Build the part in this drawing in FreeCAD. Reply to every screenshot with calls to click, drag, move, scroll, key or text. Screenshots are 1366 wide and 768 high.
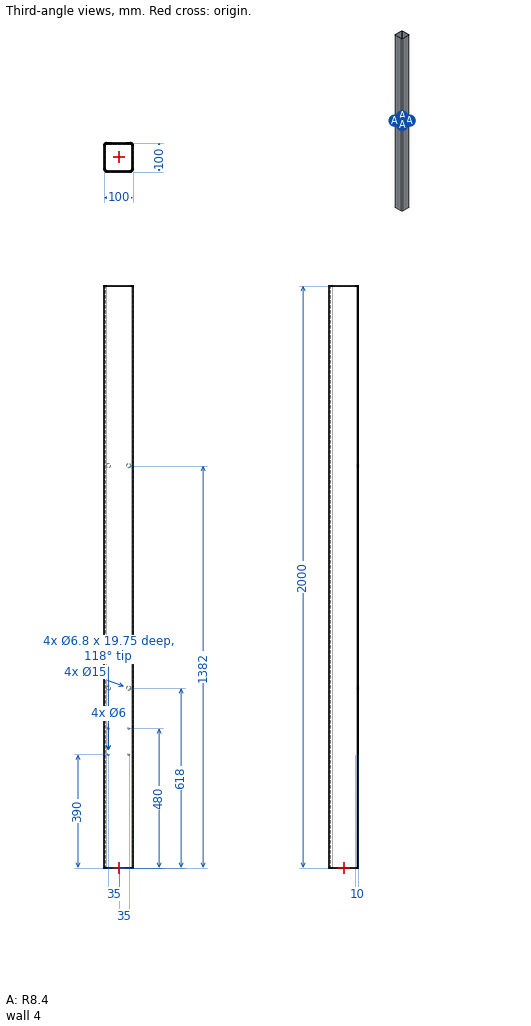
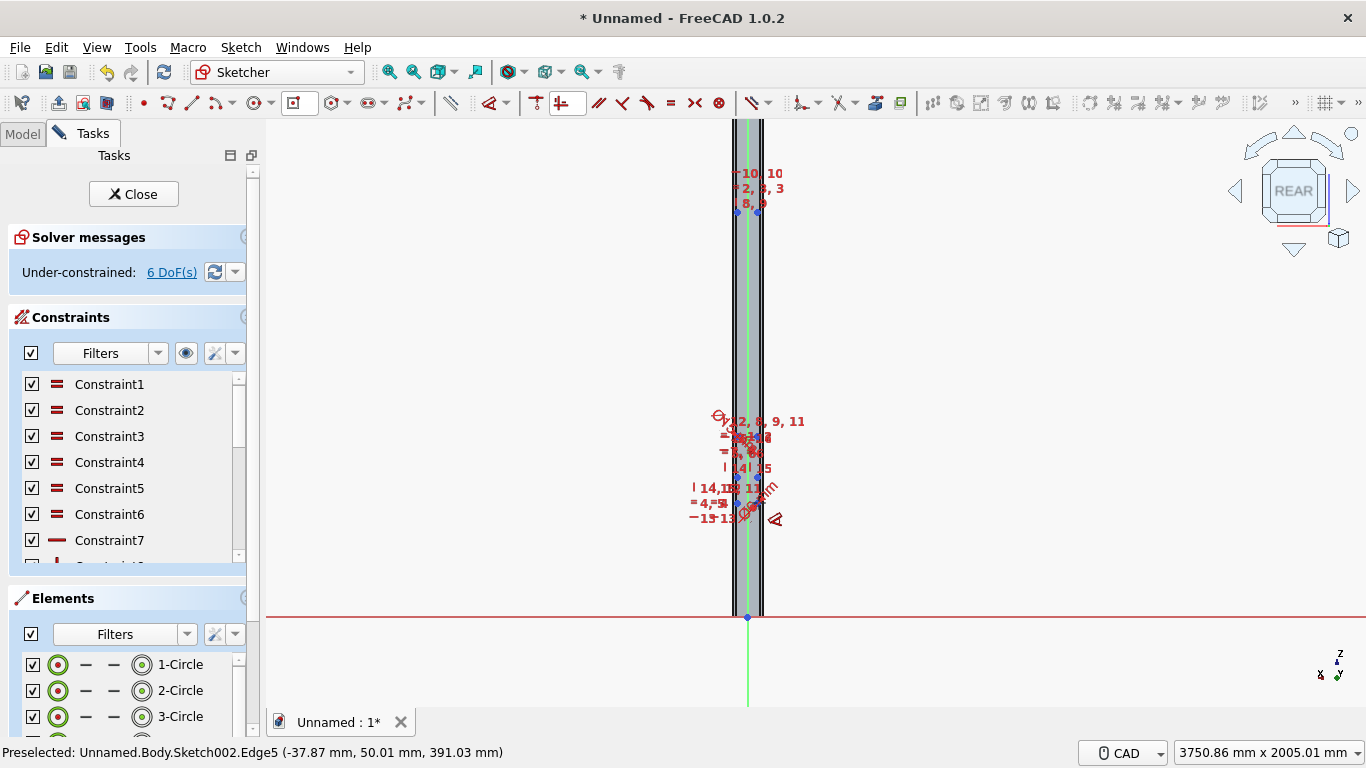
scroll(738, 437, up, 7)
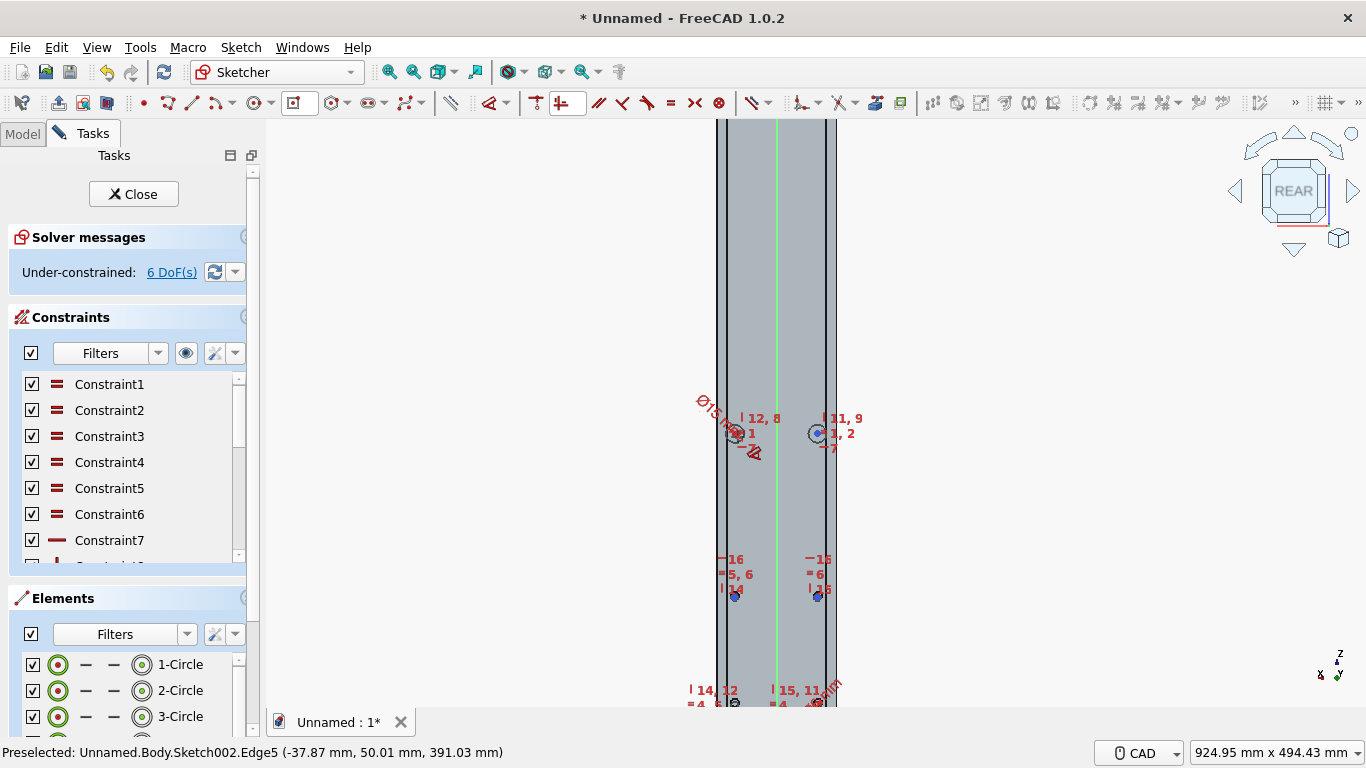
click(735, 434)
click(756, 376)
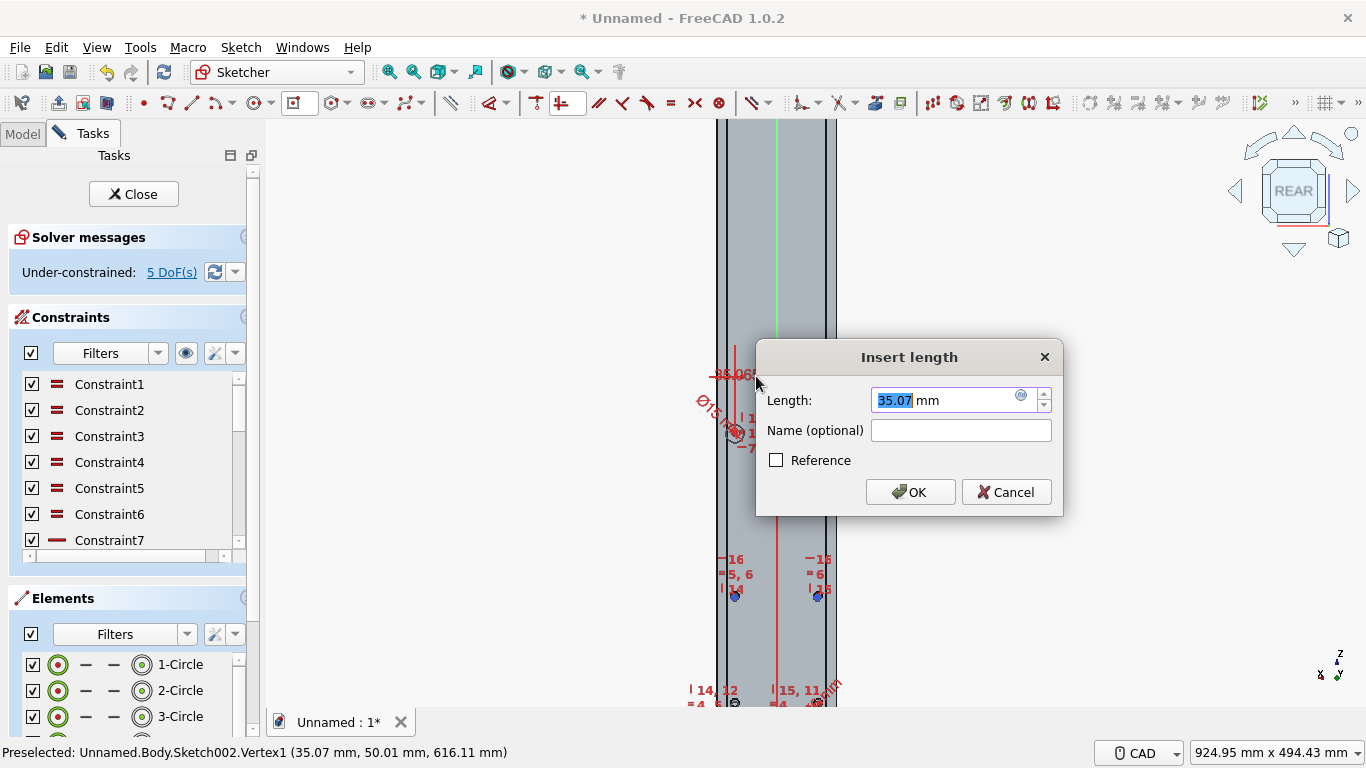
text(35)
key(Return)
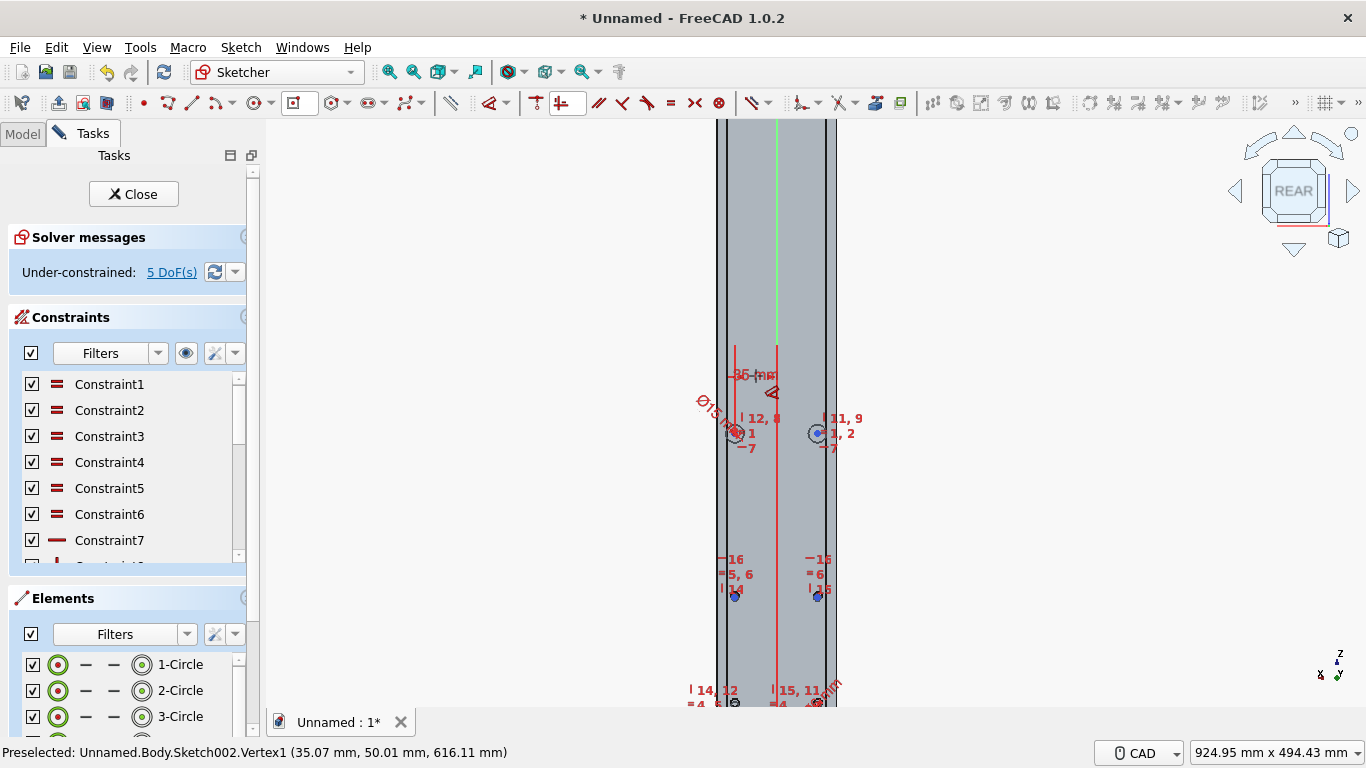
click(817, 434)
click(797, 400)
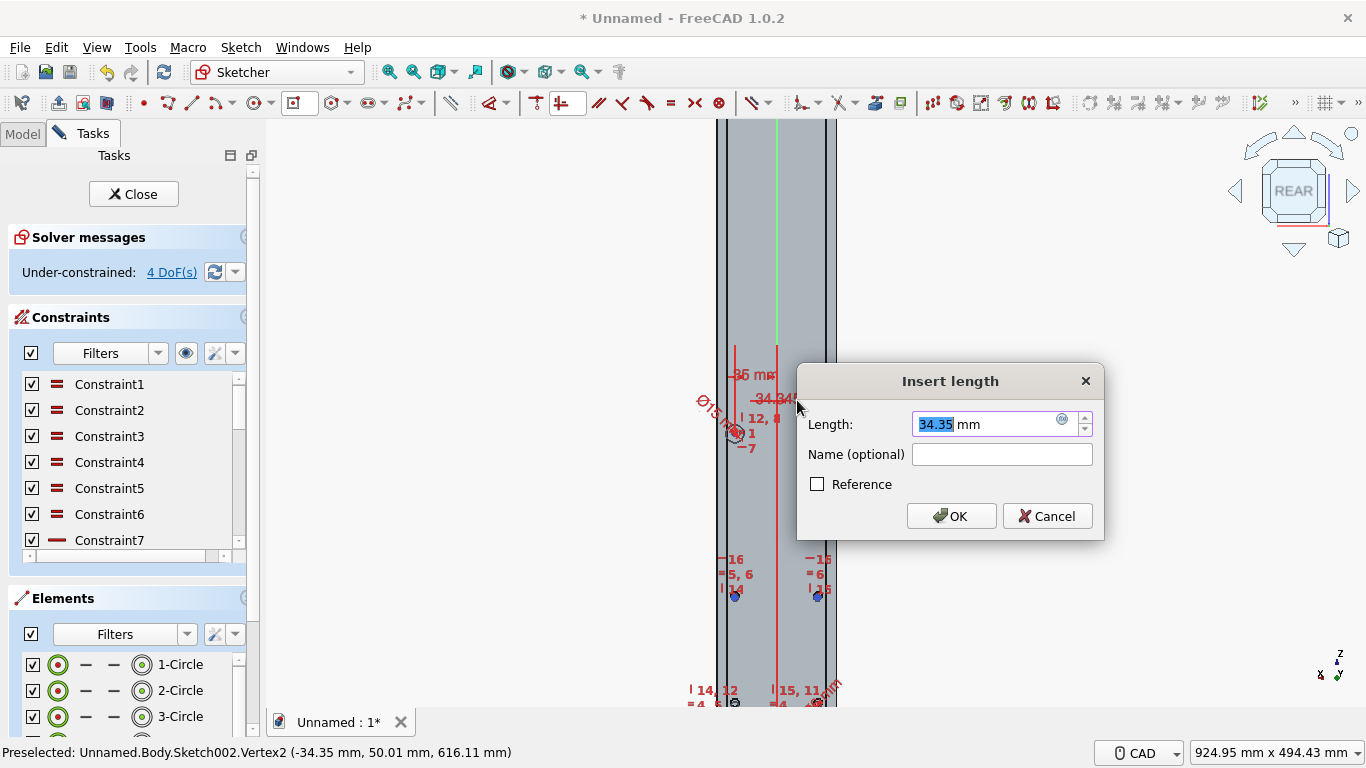
text(35)
key(Return)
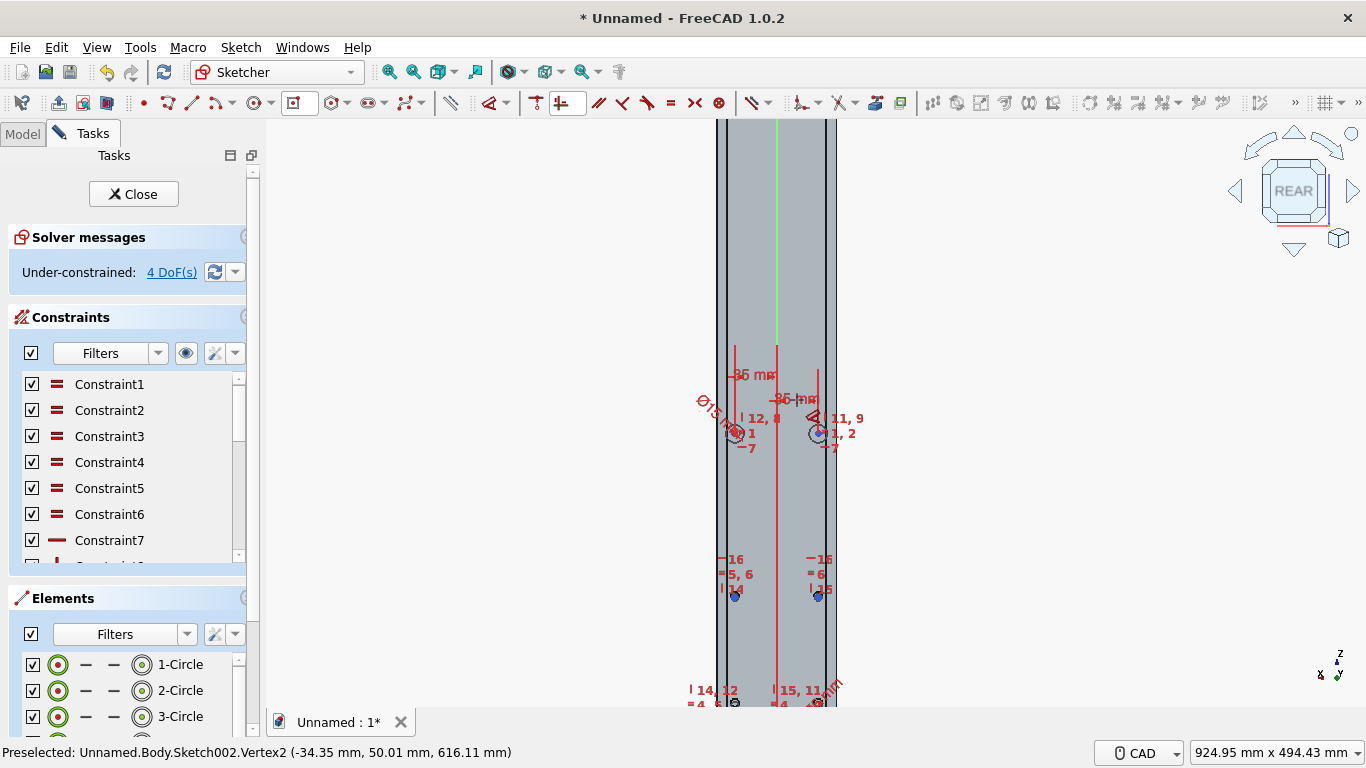
scroll(738, 437, down, 7)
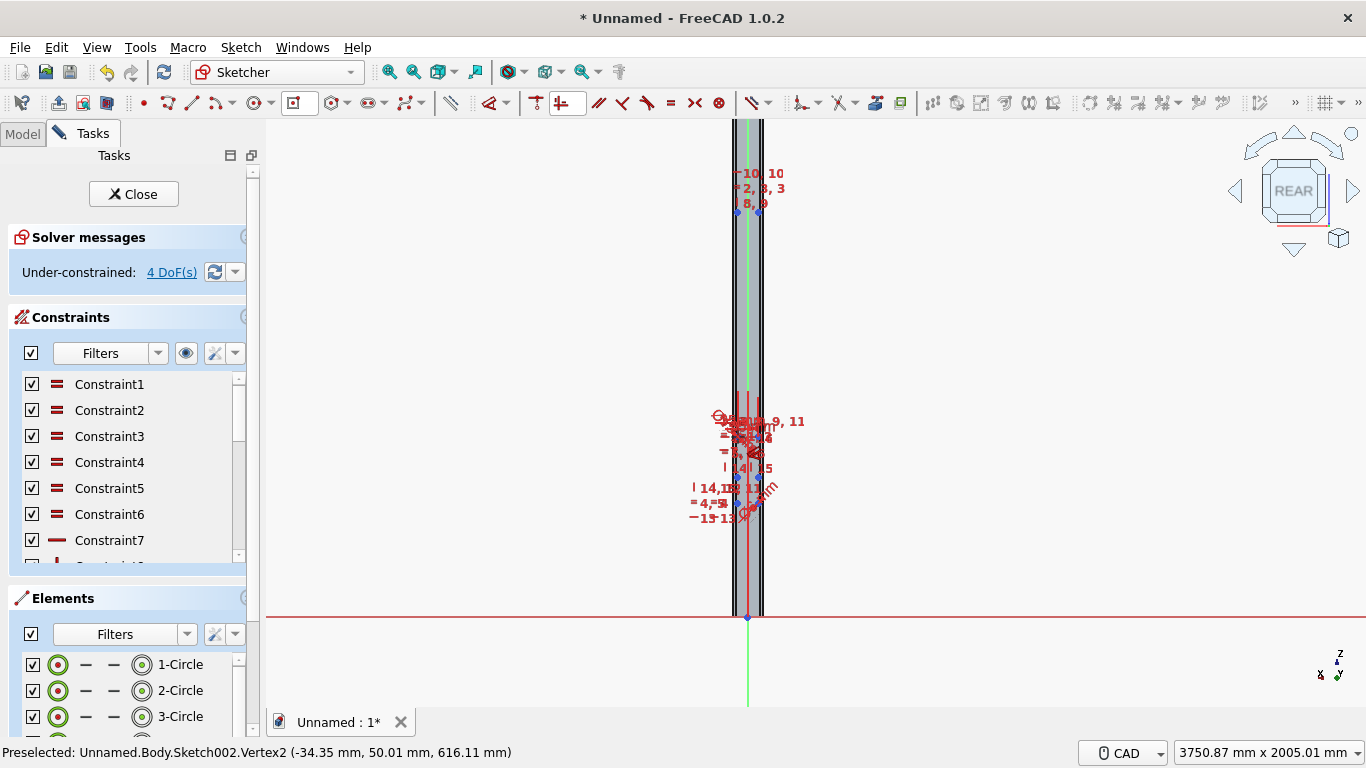
click(738, 437)
click(704, 527)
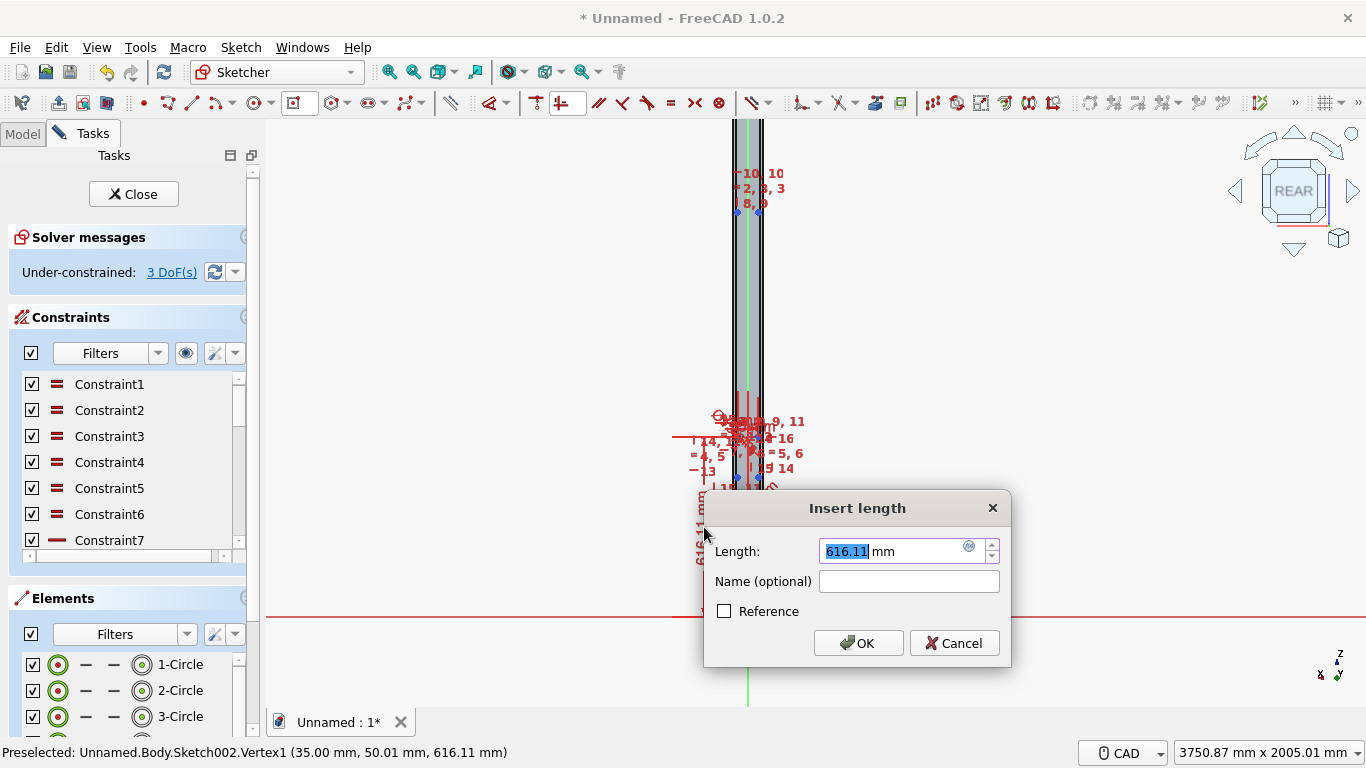
text(618)
key(Return)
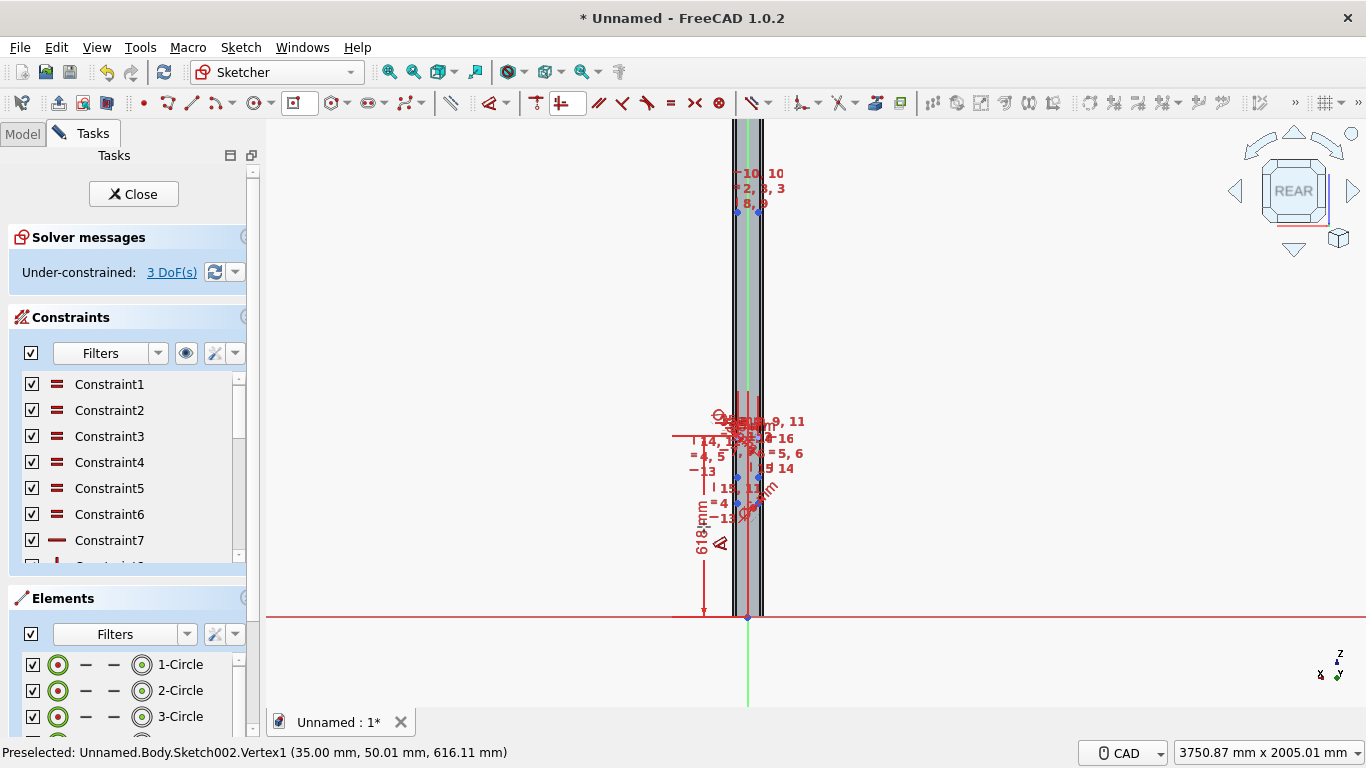
click(758, 504)
click(792, 560)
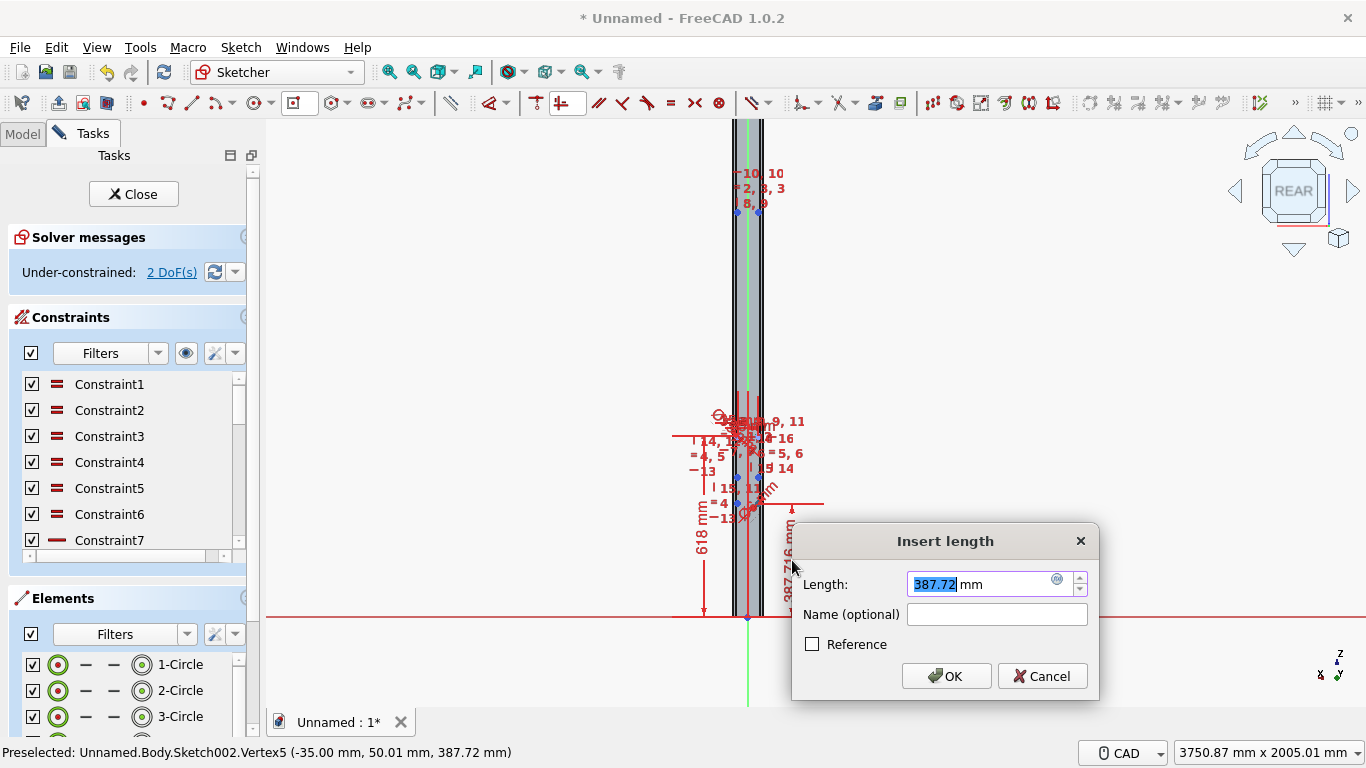
text(390)
key(Return)